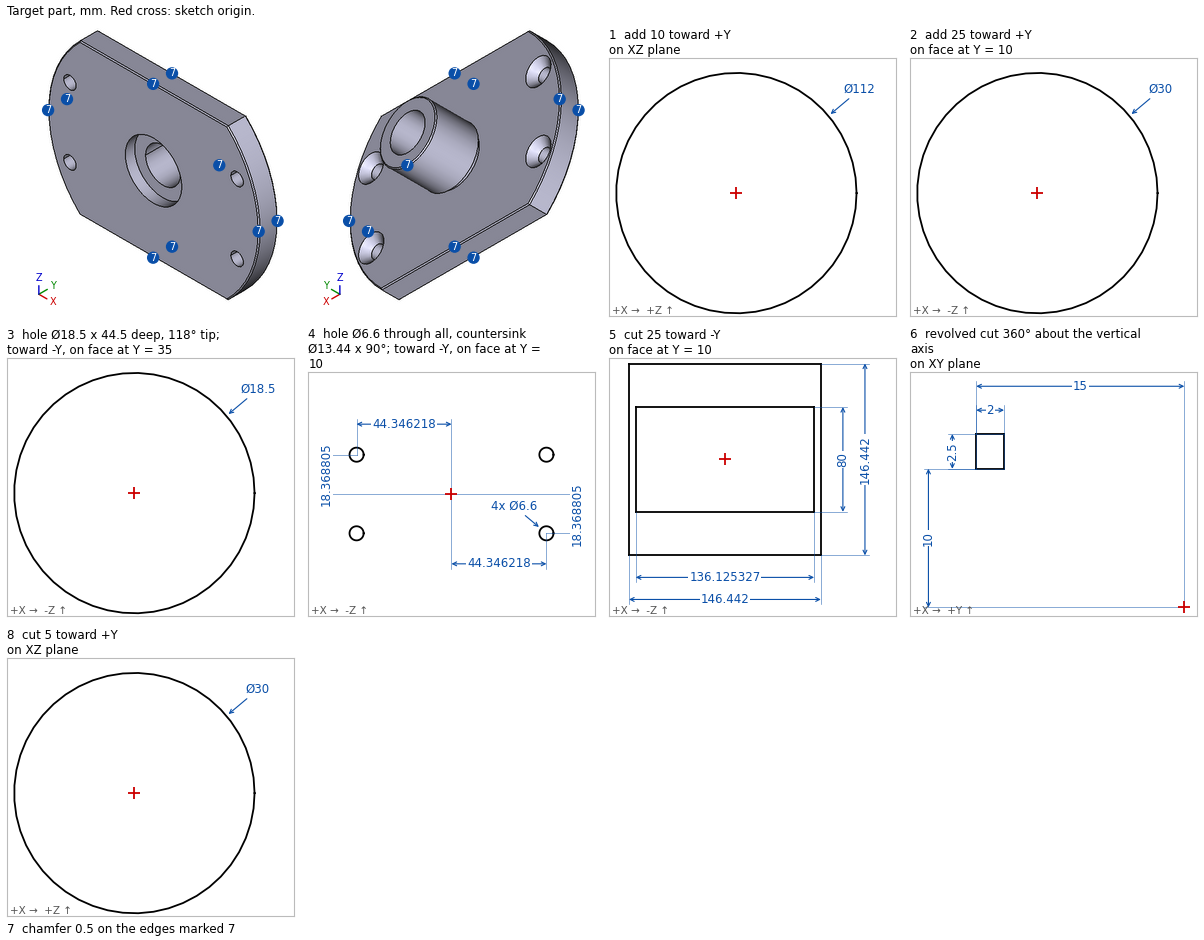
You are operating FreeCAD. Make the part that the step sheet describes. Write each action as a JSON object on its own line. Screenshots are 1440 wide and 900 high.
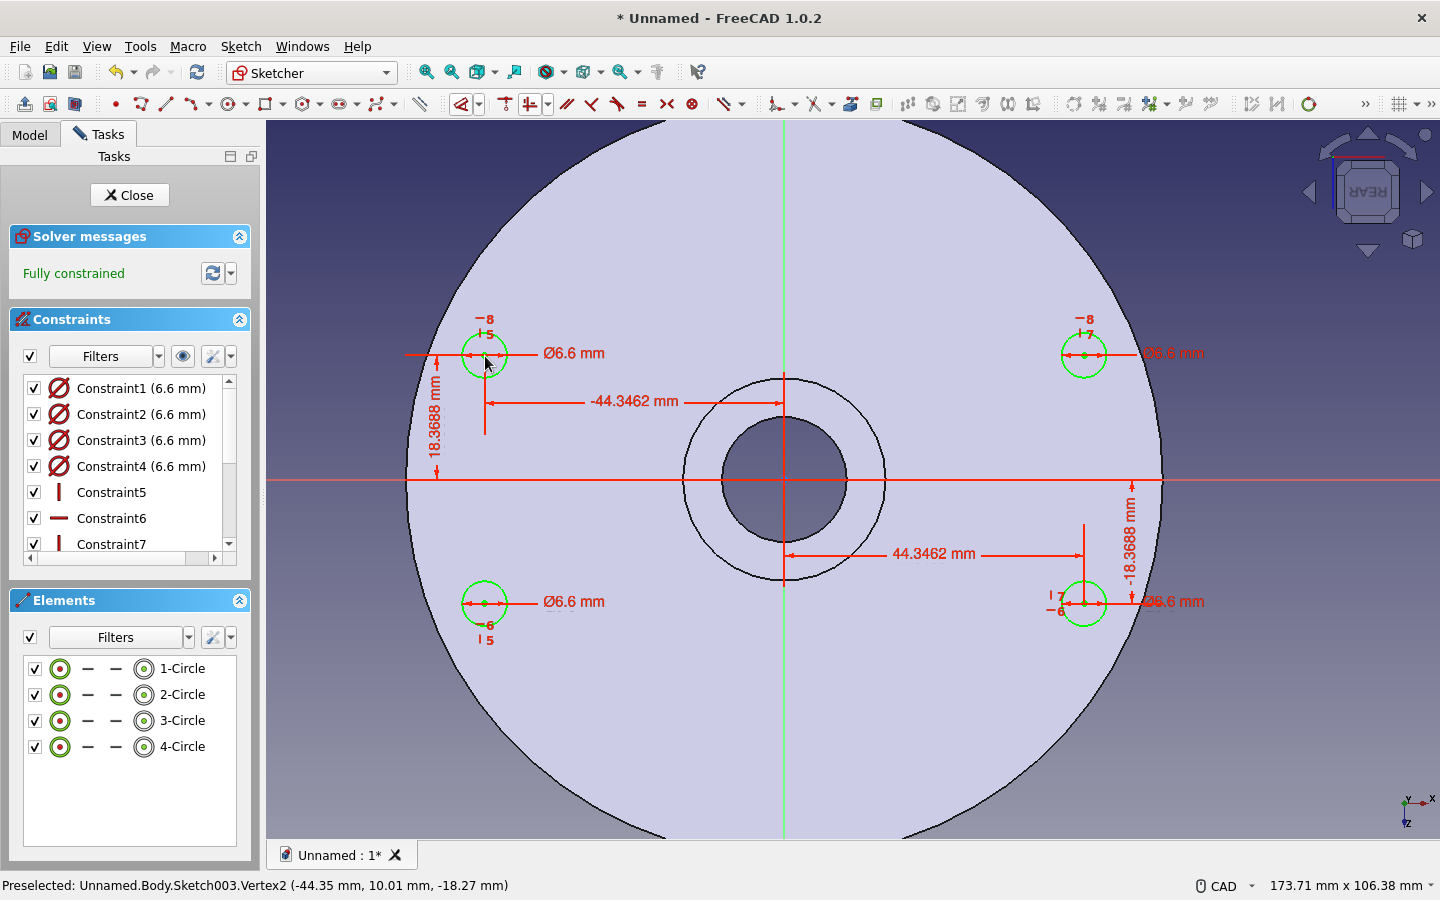
{"action": "left_click", "coordinate": [130, 195]}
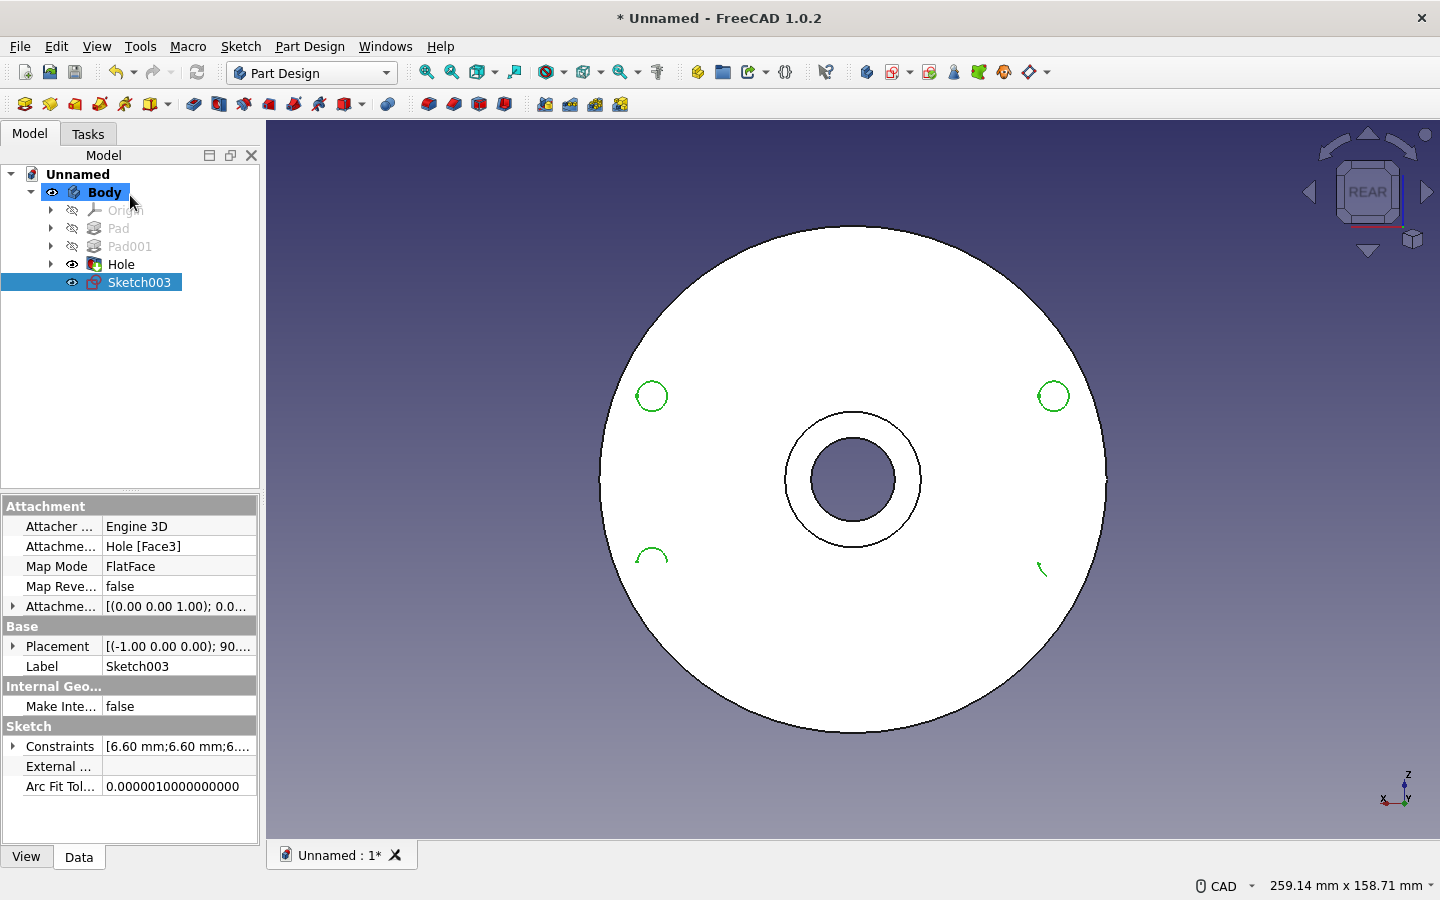
{"action": "left_click", "coordinate": [219, 104]}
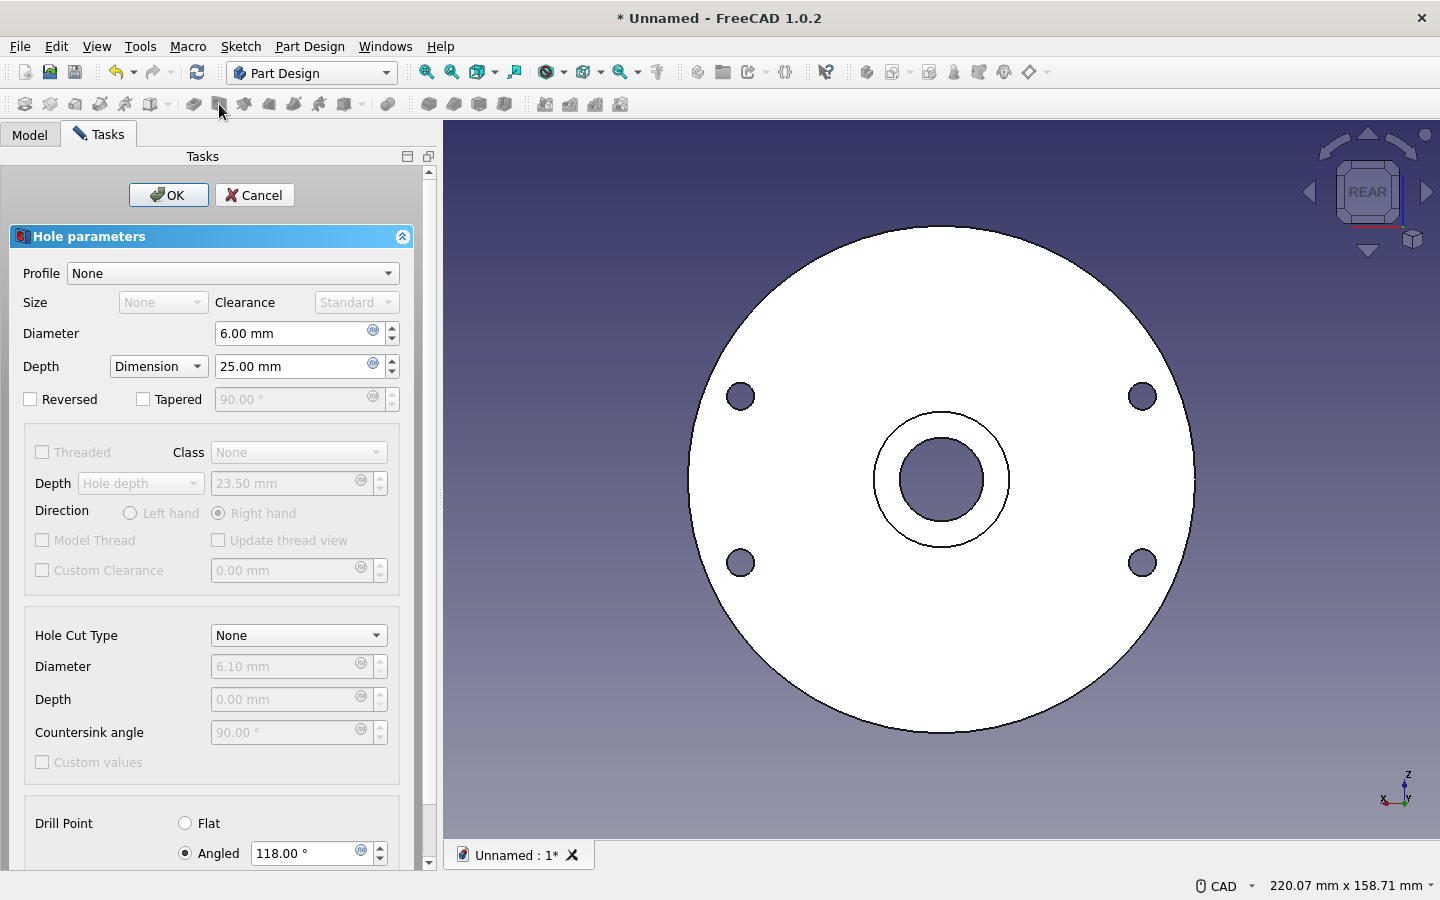
{"action": "triple_click", "coordinate": [300, 334]}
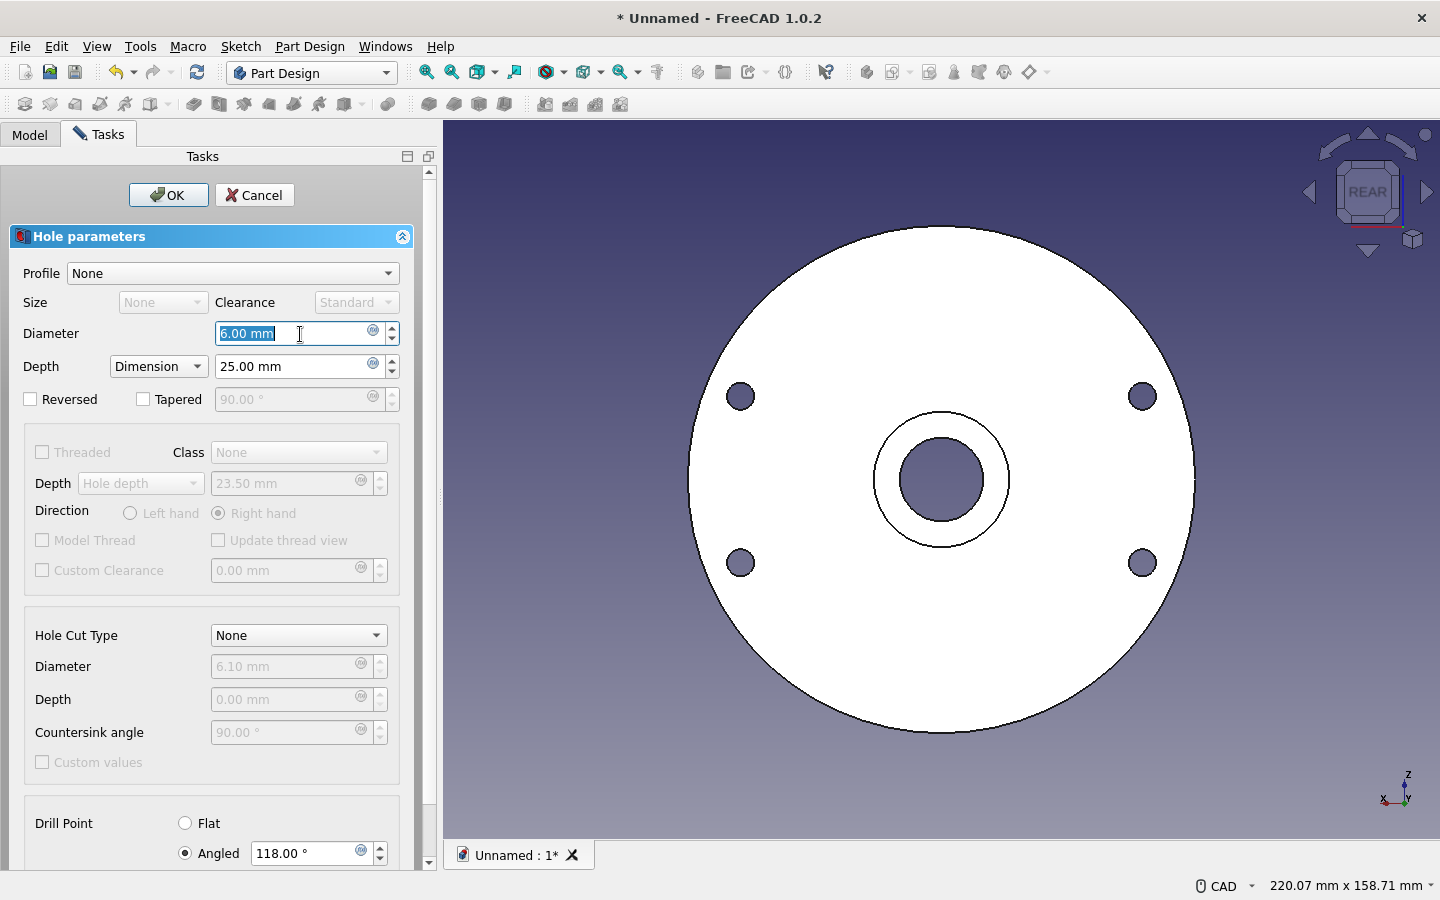
{"action": "type", "text": "6.6"}
{"action": "key", "text": "Tab"}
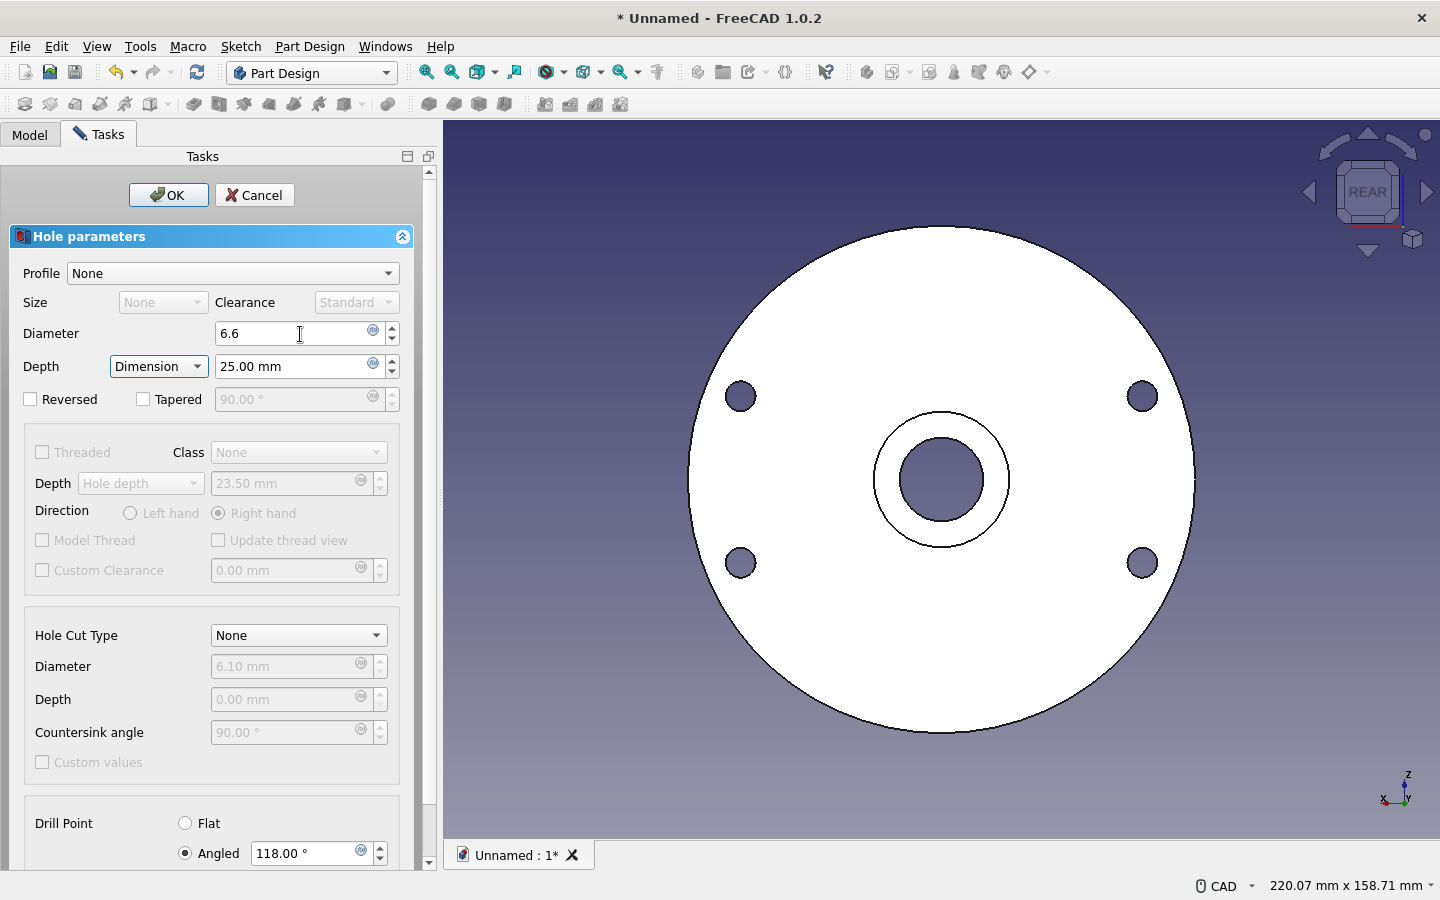
{"action": "left_click", "coordinate": [160, 366]}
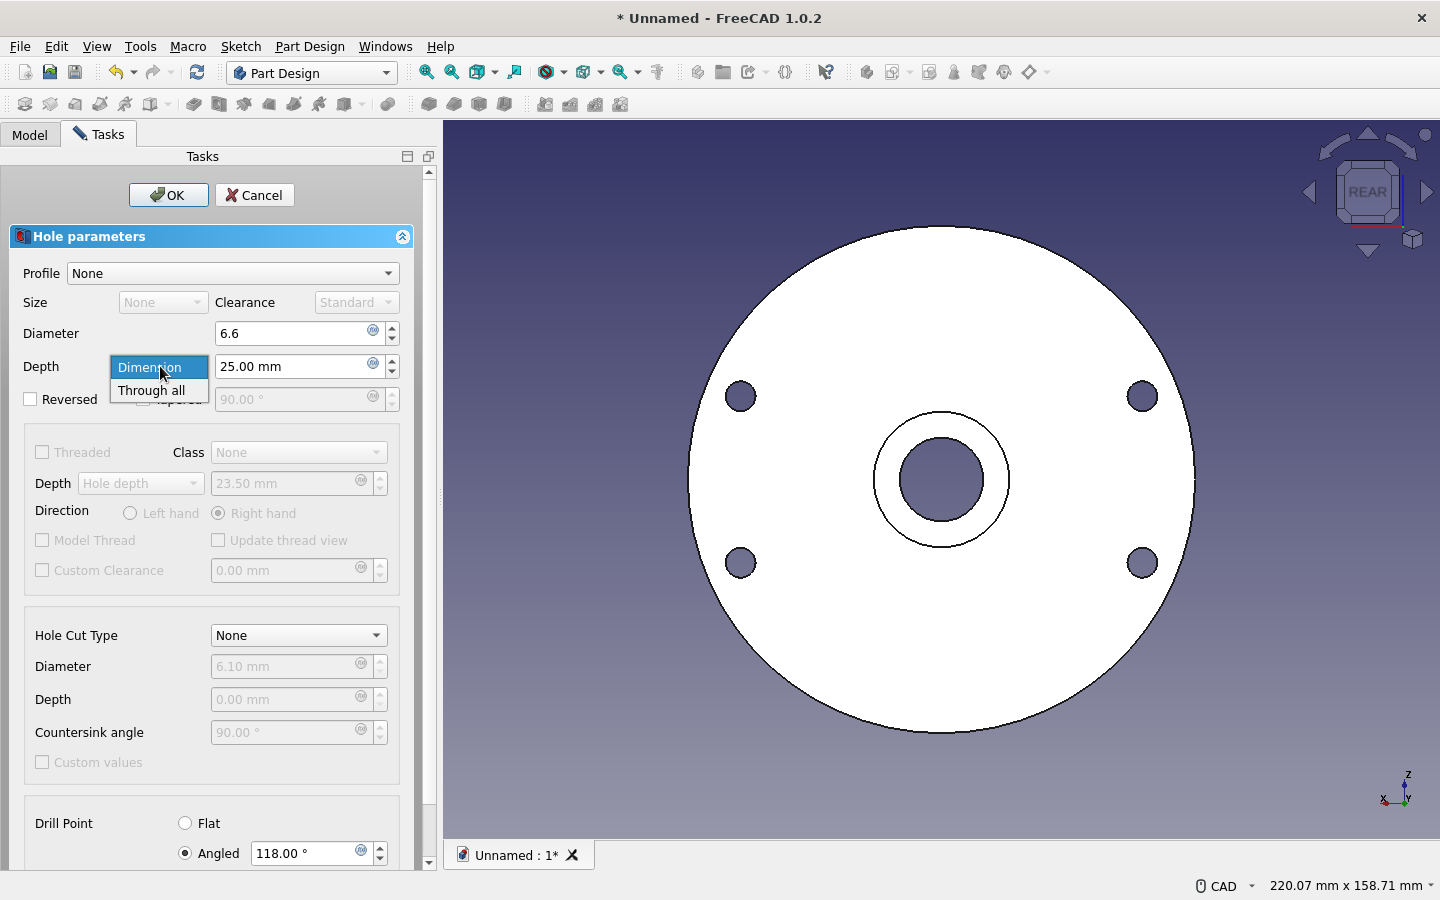
{"action": "left_click", "coordinate": [158, 390]}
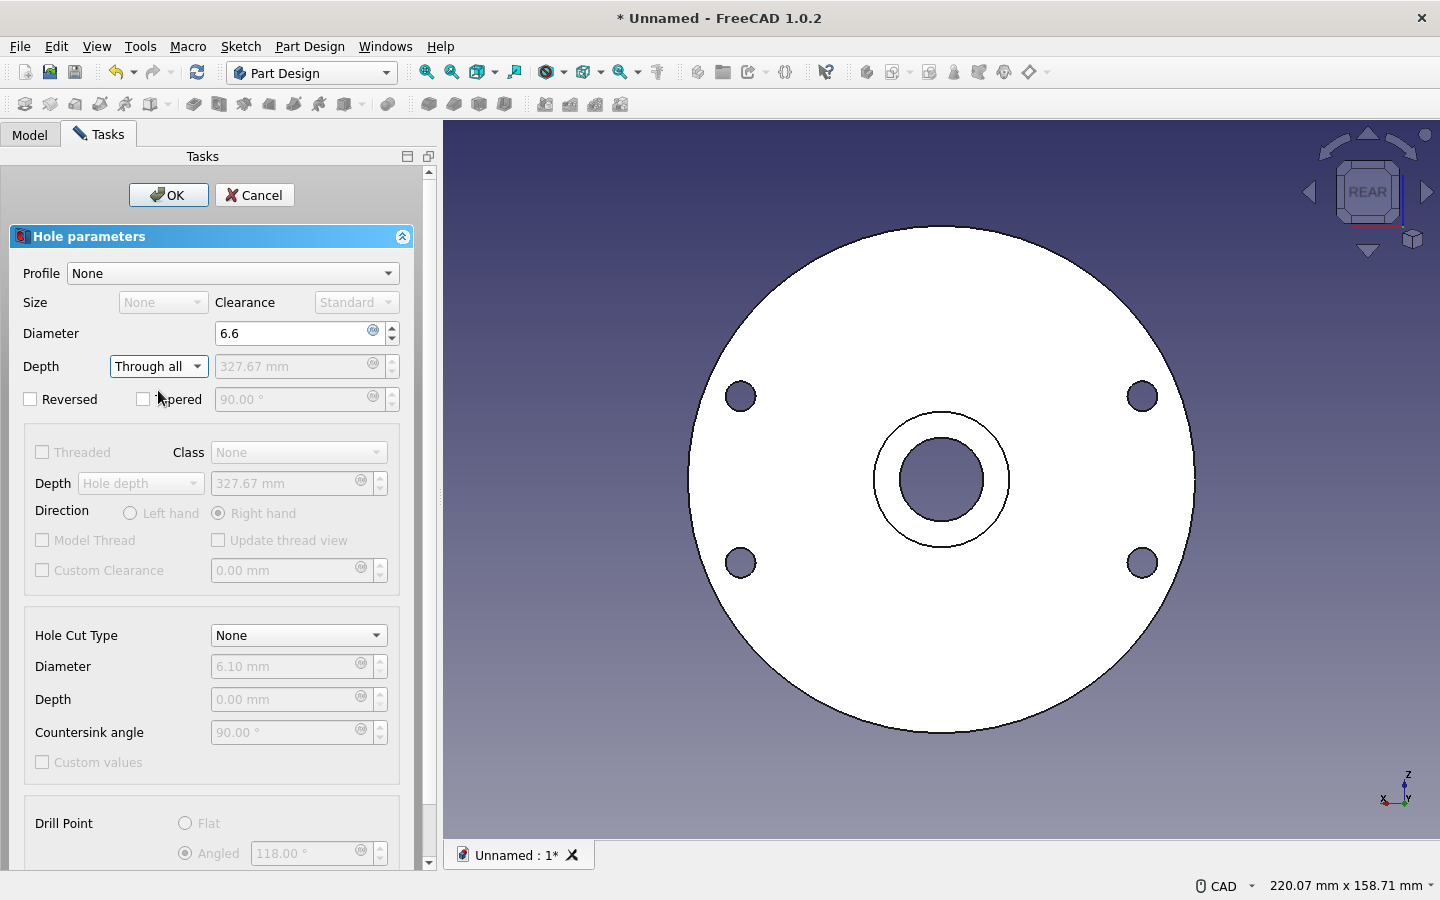
{"action": "left_click", "coordinate": [300, 636]}